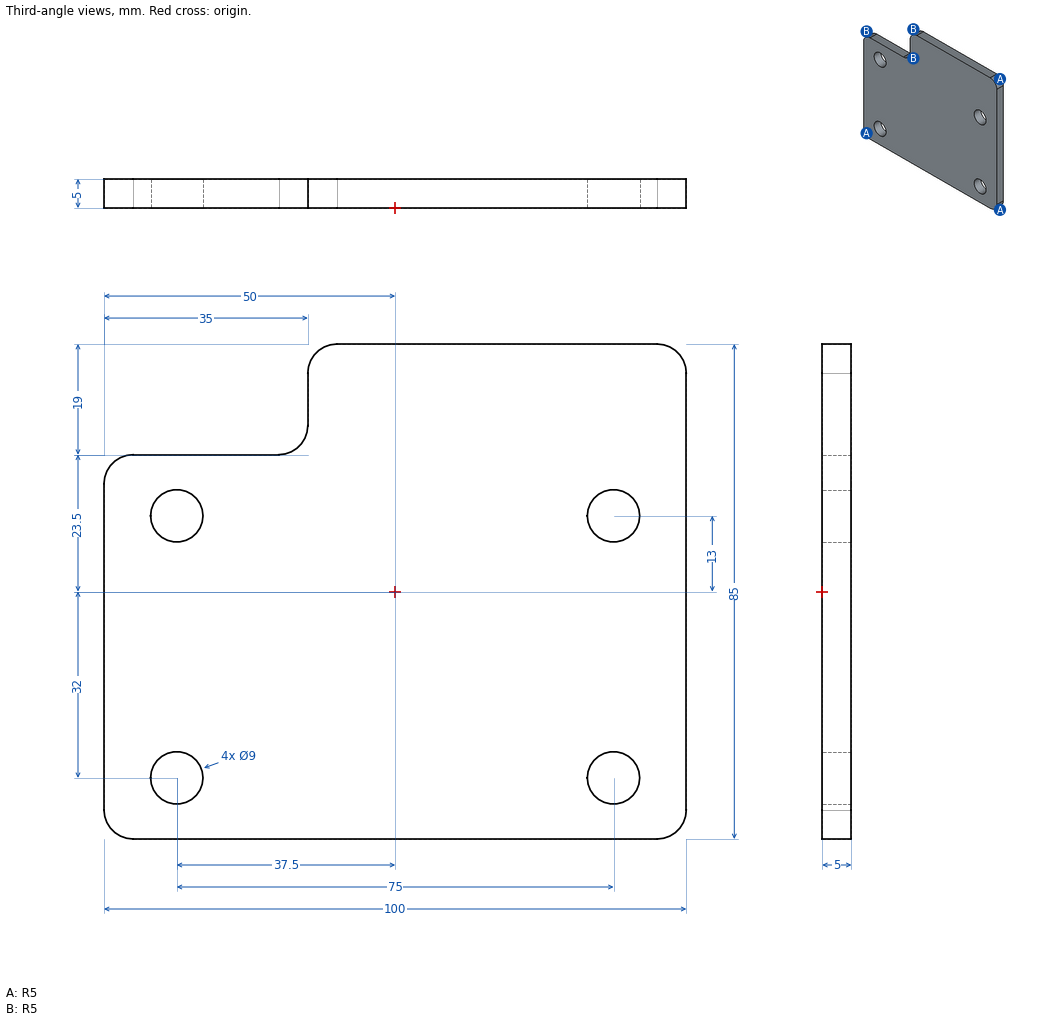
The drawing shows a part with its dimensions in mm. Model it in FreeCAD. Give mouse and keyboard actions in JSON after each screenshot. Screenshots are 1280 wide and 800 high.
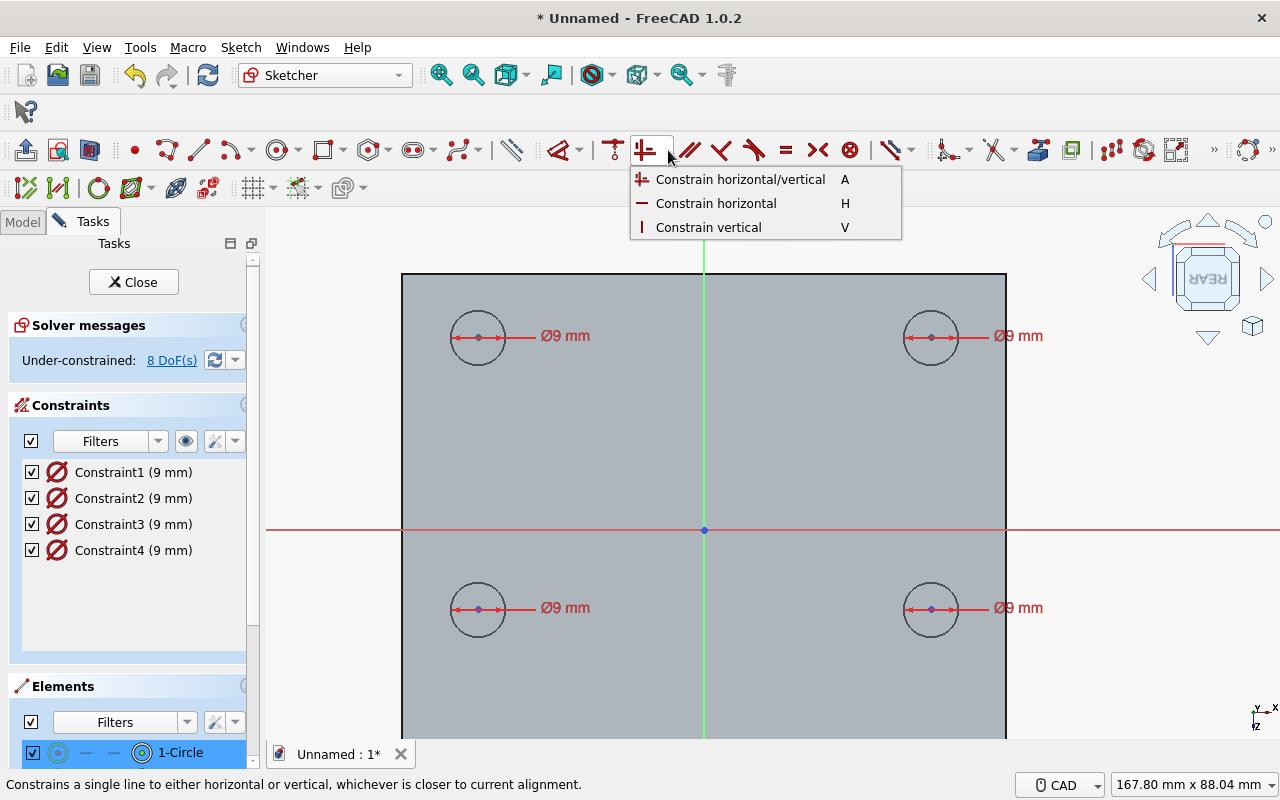
{"action": "left_click", "coordinate": [766, 203]}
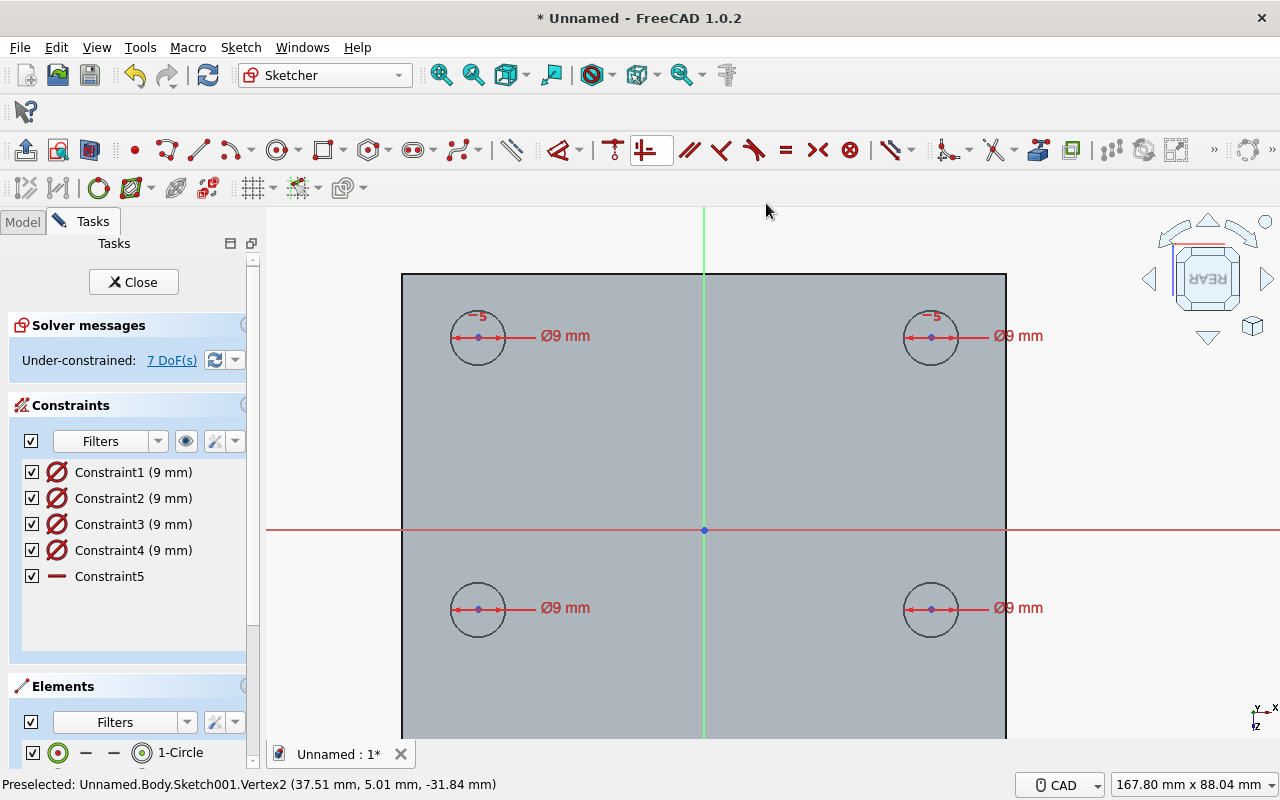
{"action": "left_click", "coordinate": [931, 338]}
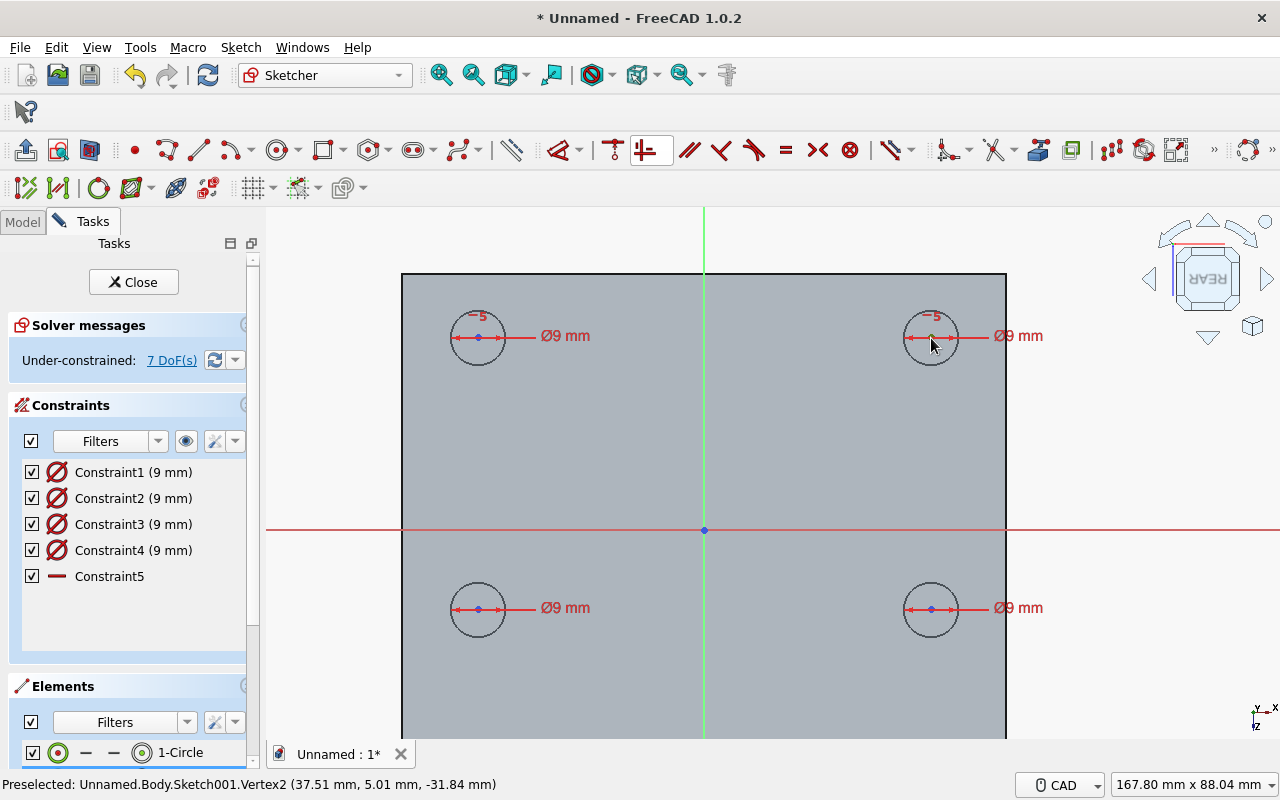
{"action": "left_click", "coordinate": [931, 610]}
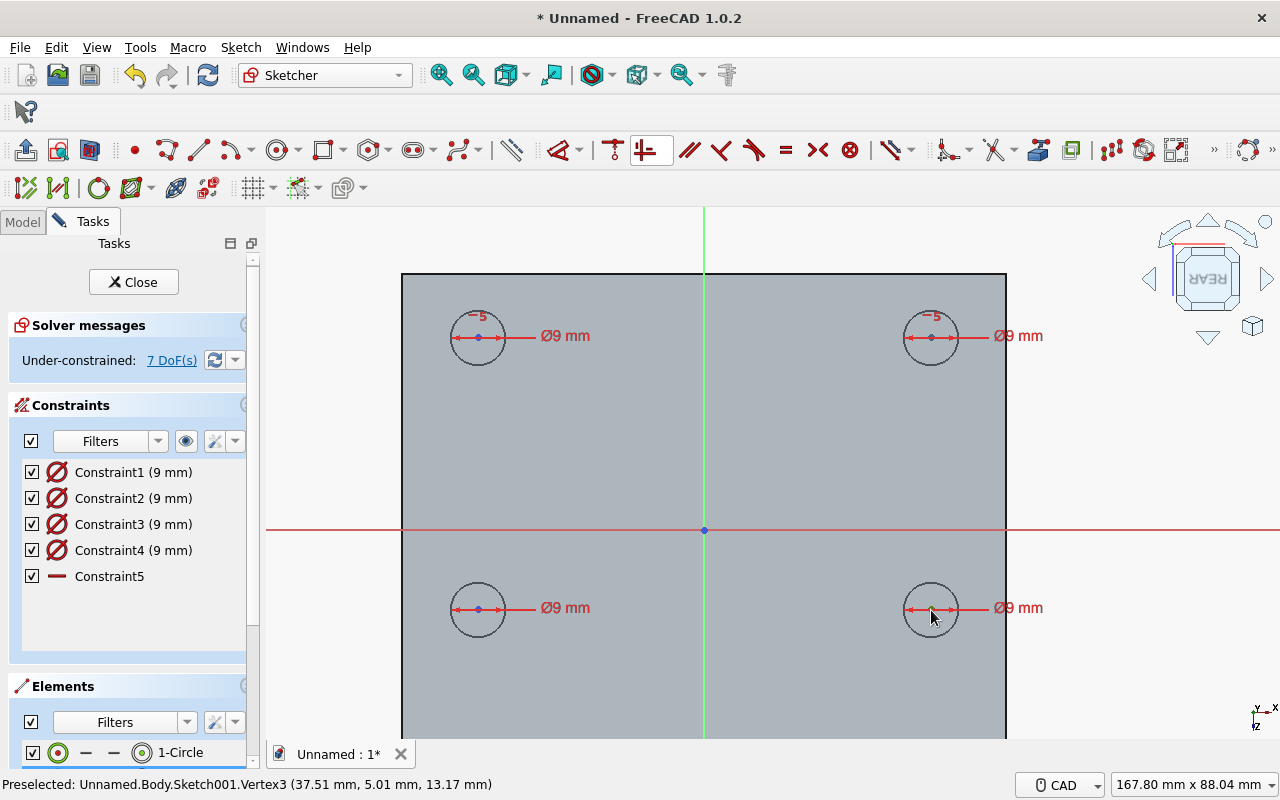
{"action": "left_click", "coordinate": [668, 150]}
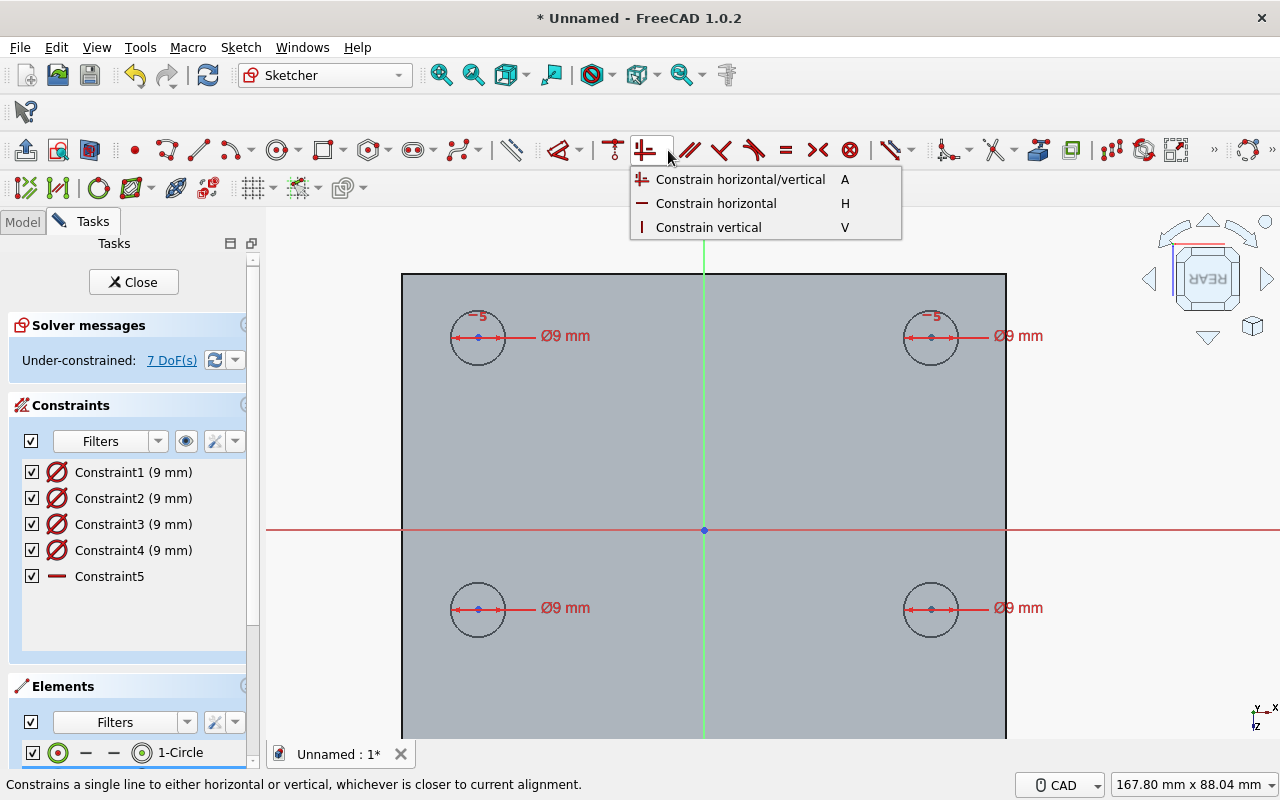
{"action": "left_click", "coordinate": [766, 227]}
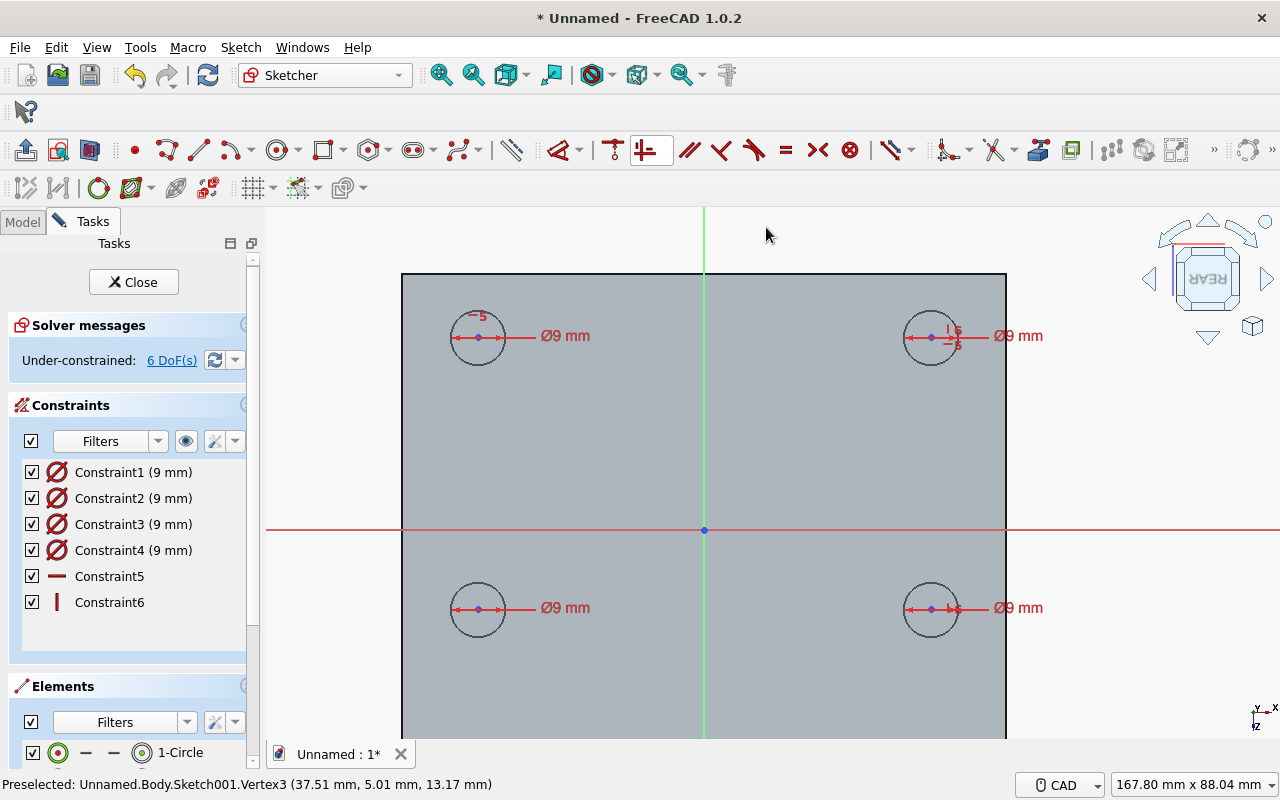
{"action": "left_click", "coordinate": [478, 338]}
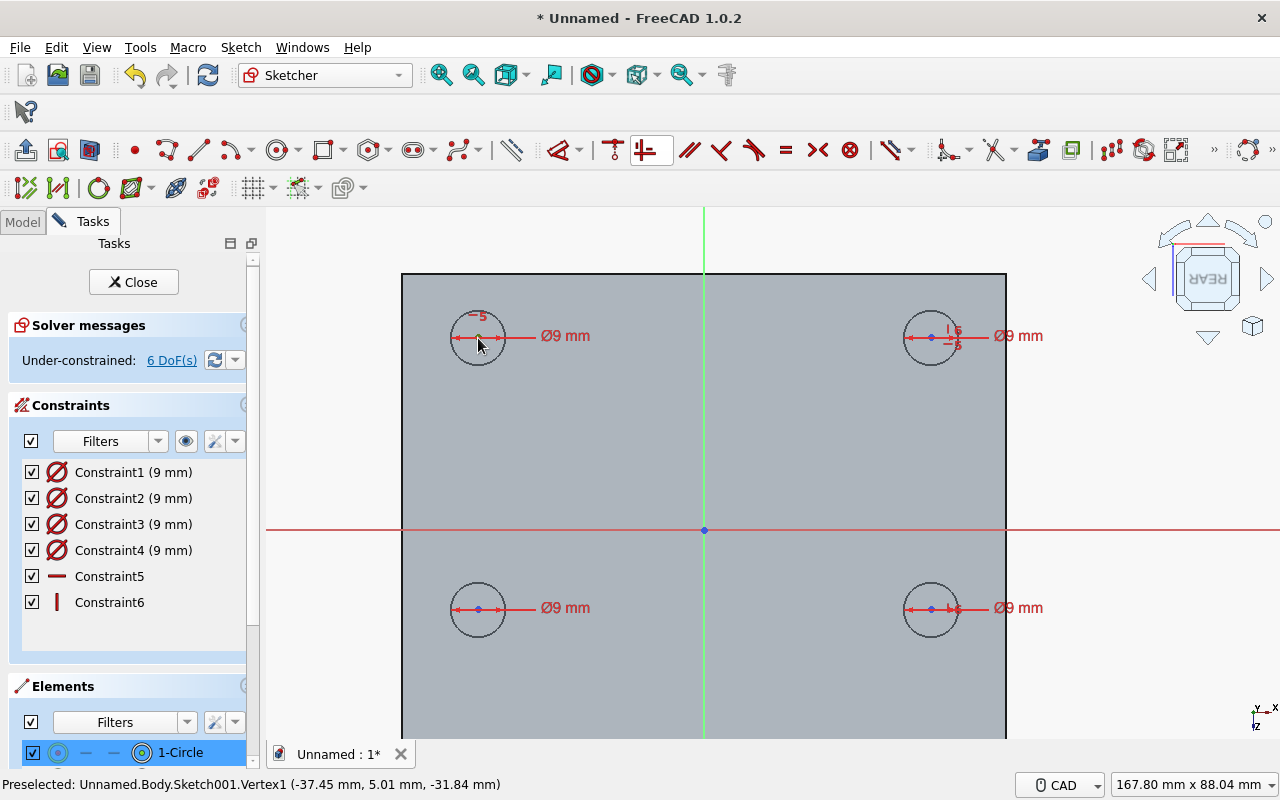
{"action": "left_click", "coordinate": [478, 610]}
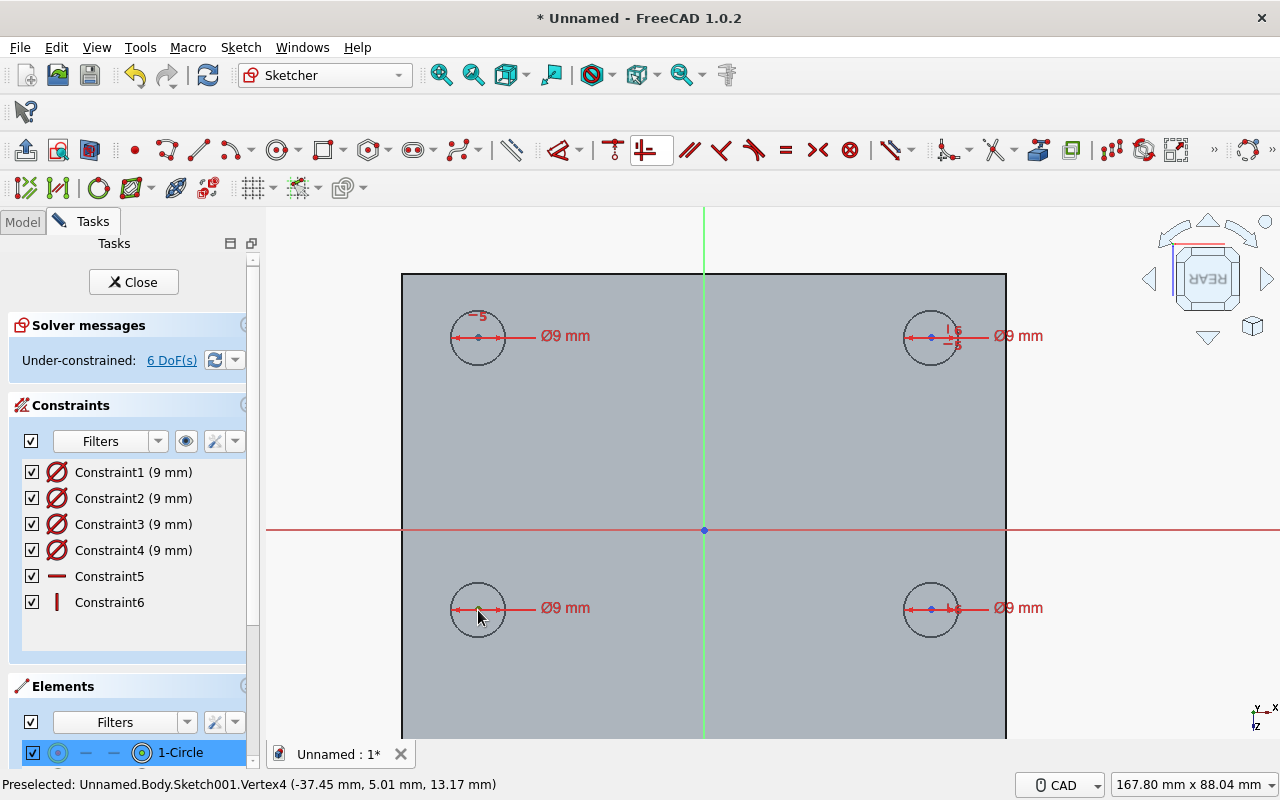
{"action": "left_click", "coordinate": [668, 150]}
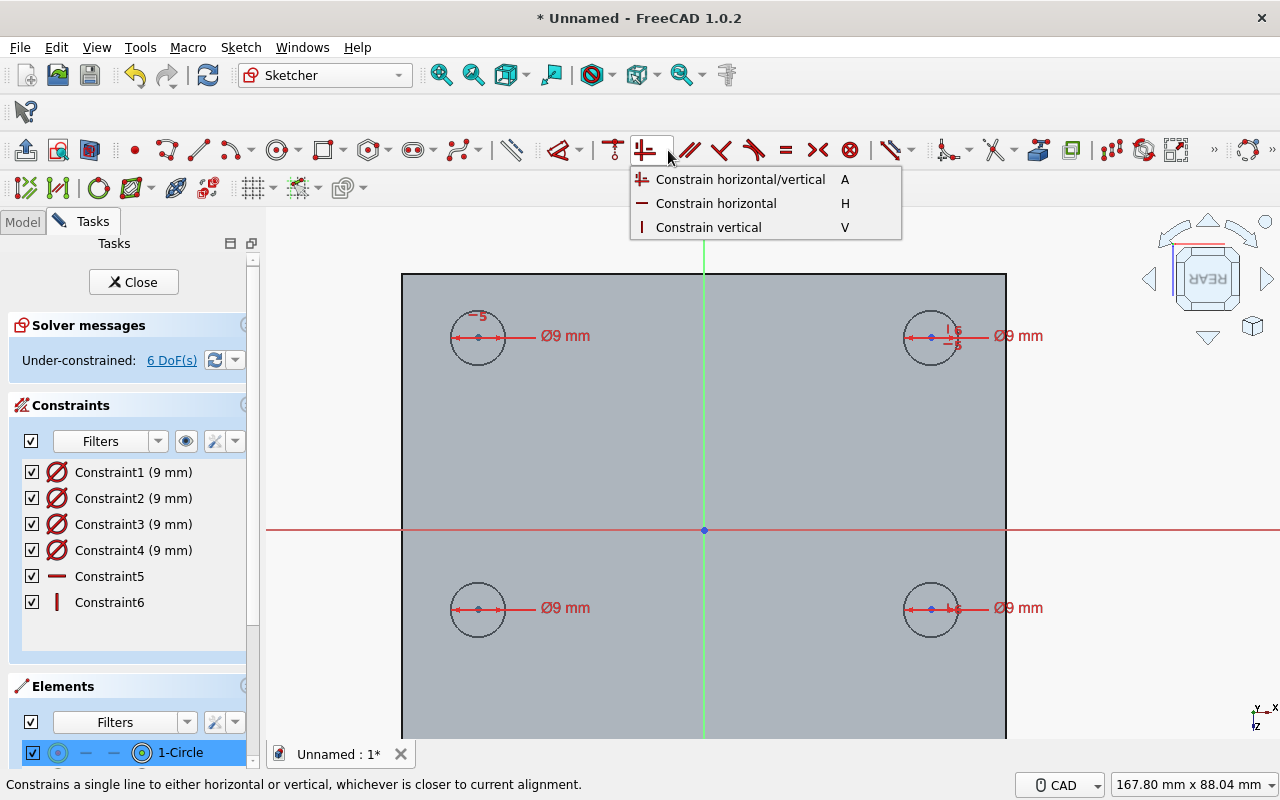
{"action": "left_click", "coordinate": [766, 227]}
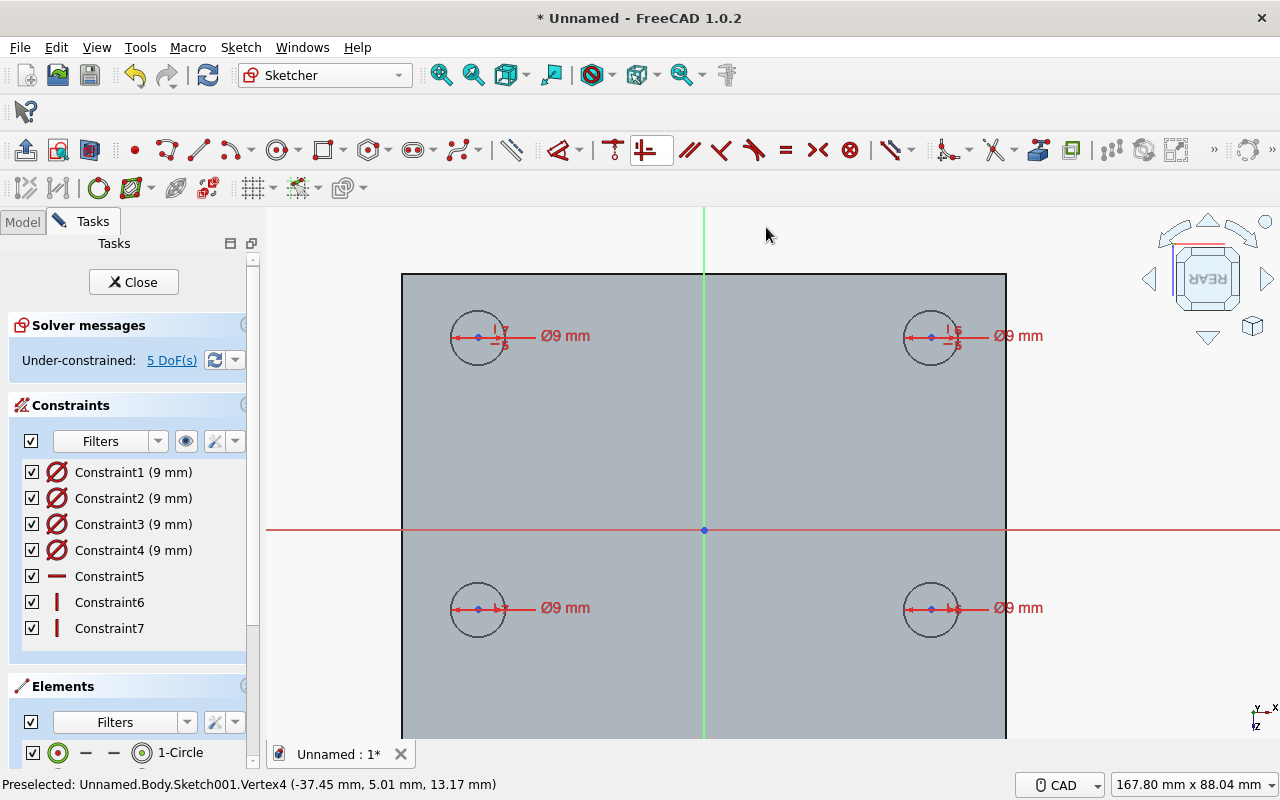
{"action": "left_click", "coordinate": [931, 610]}